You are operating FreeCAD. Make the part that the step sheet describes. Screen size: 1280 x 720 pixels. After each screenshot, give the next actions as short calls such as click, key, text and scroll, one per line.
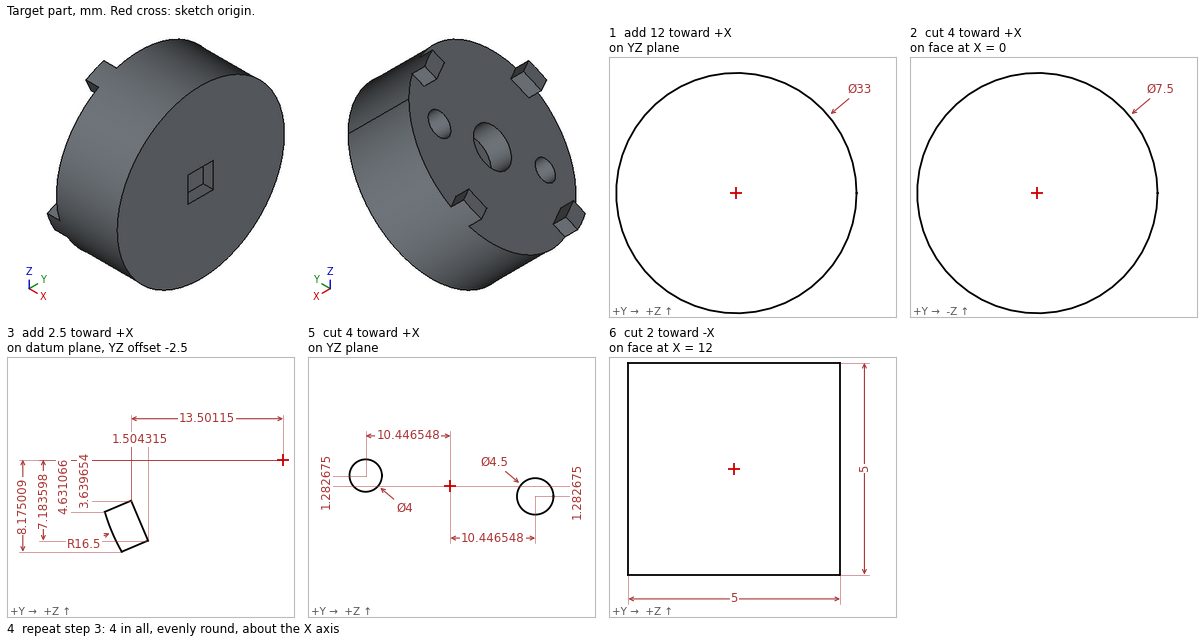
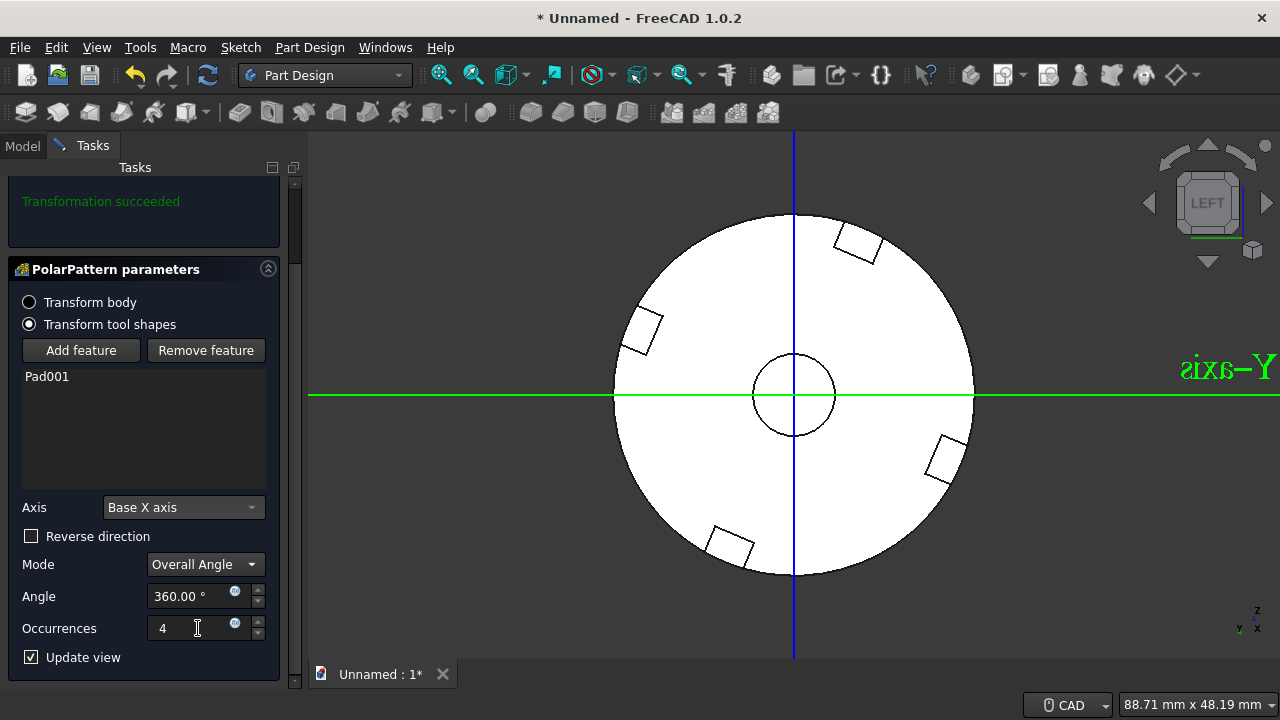
scroll(295, 432, up, 3)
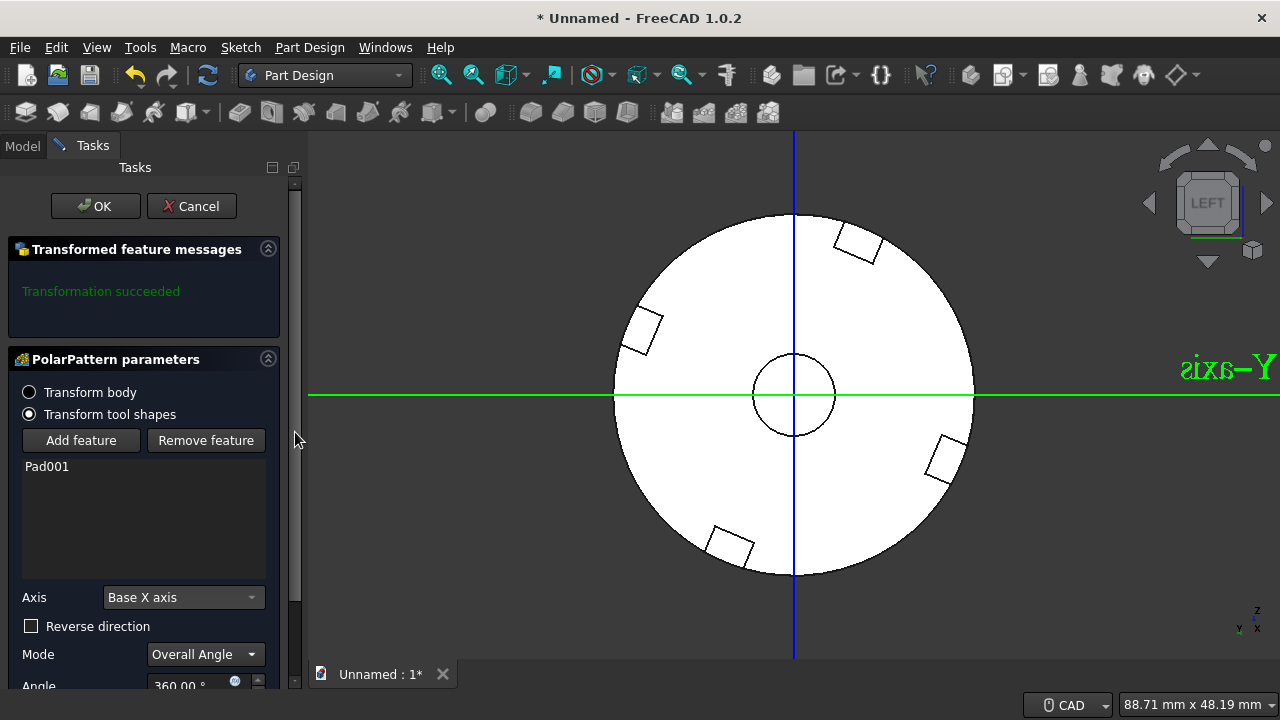
click(96, 206)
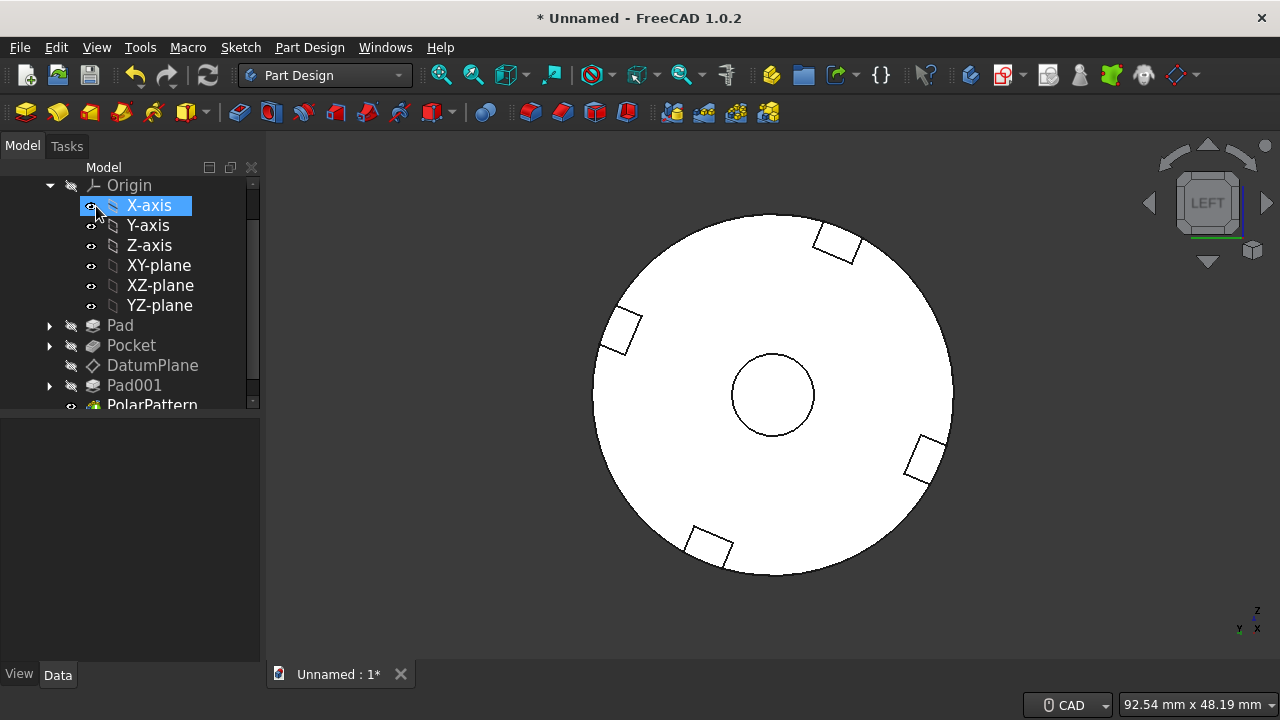
click(1004, 76)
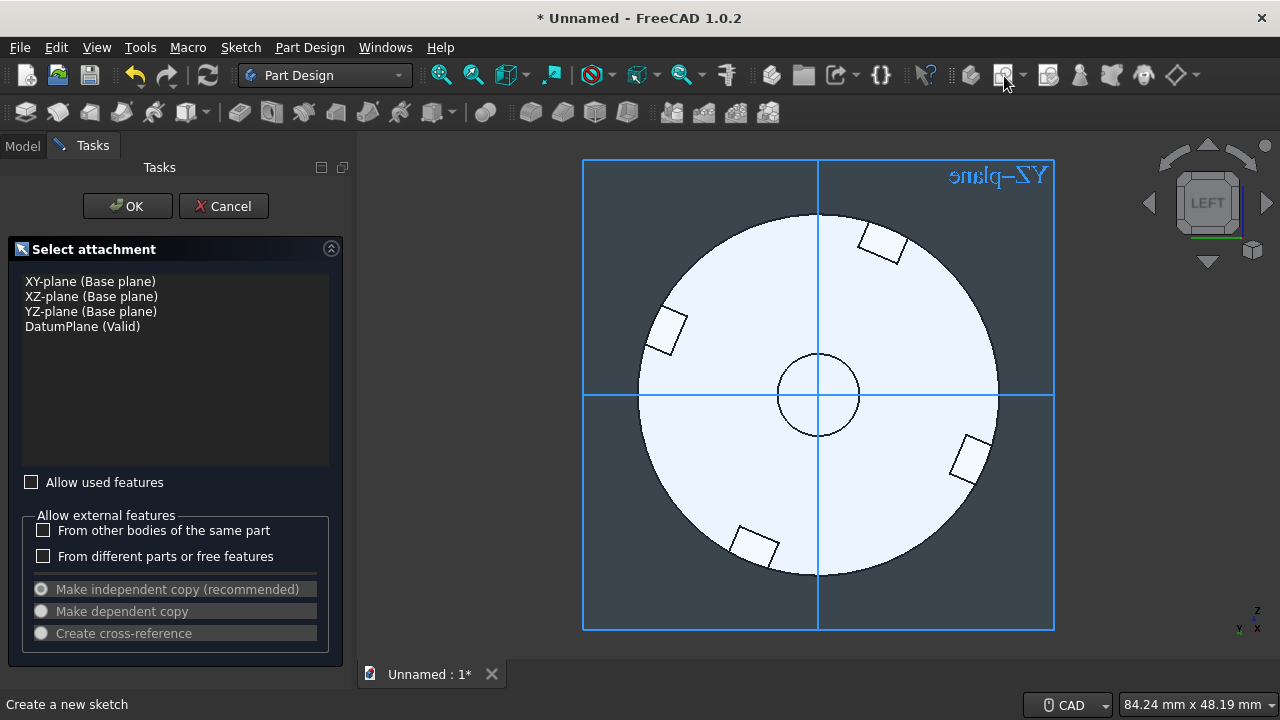
click(82, 312)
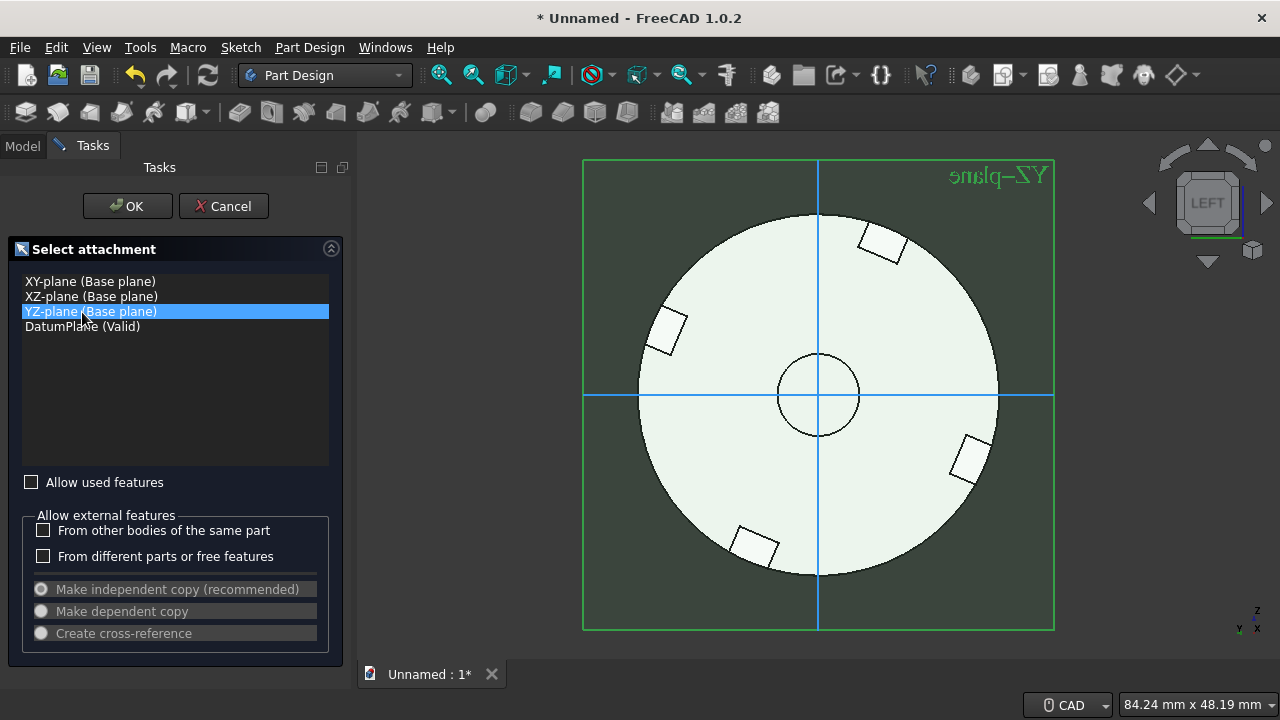
click(128, 206)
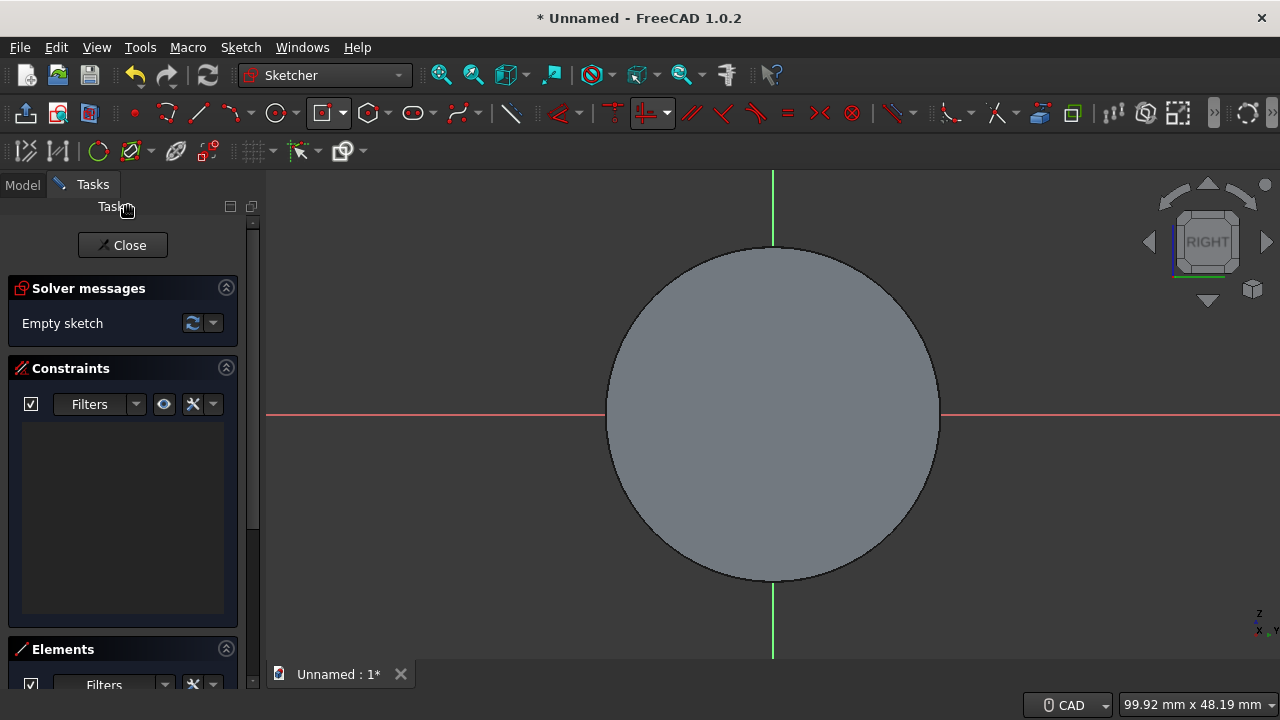
key(q)
key(s)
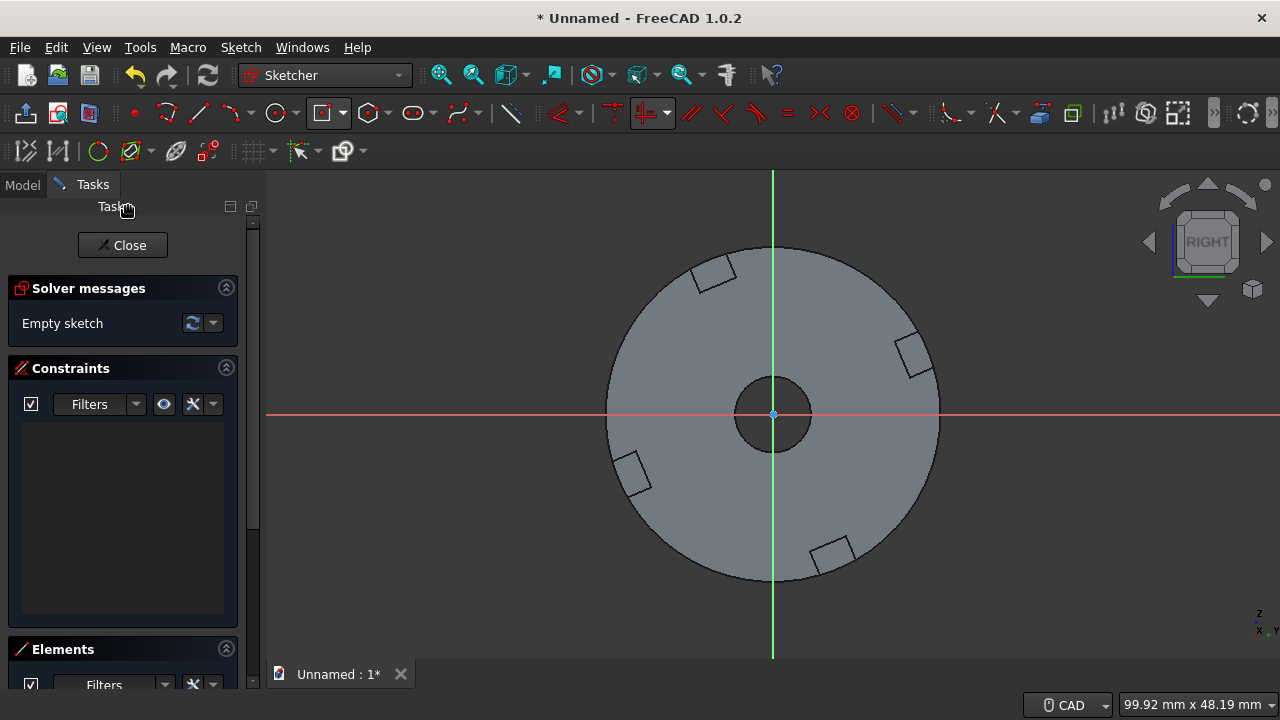
scroll(831, 417, up, 4)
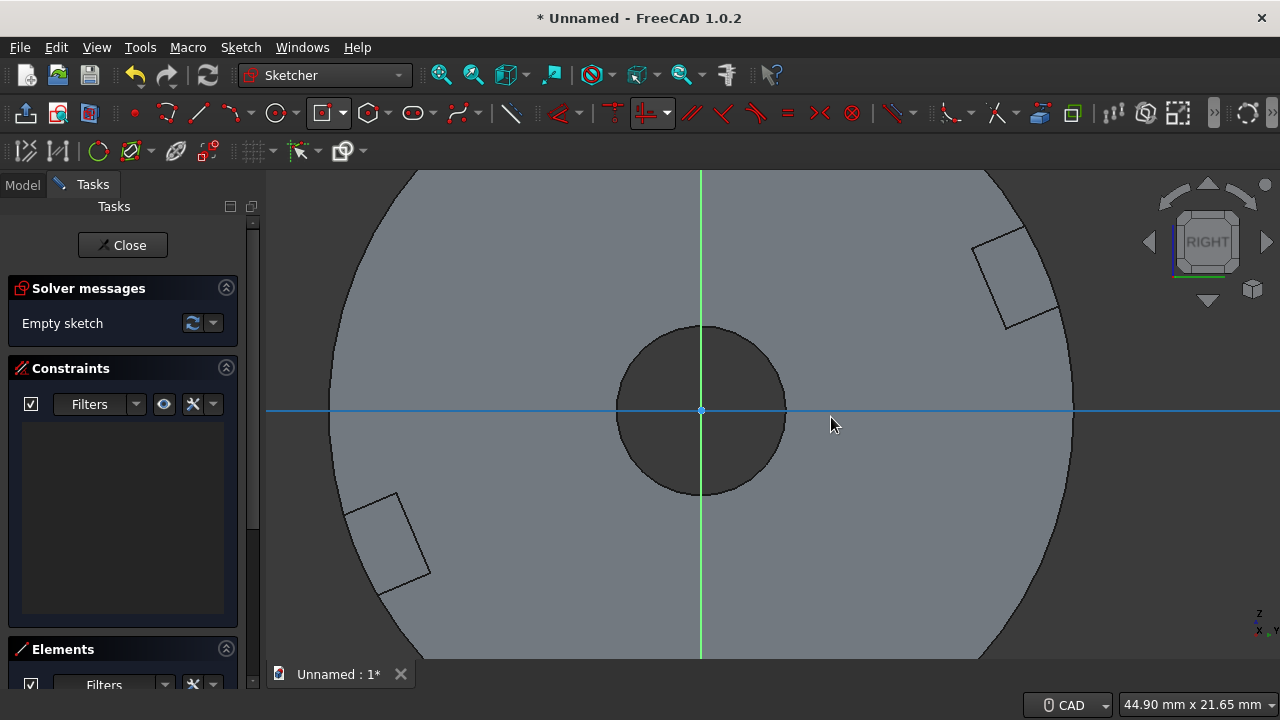
key(g)
key(c)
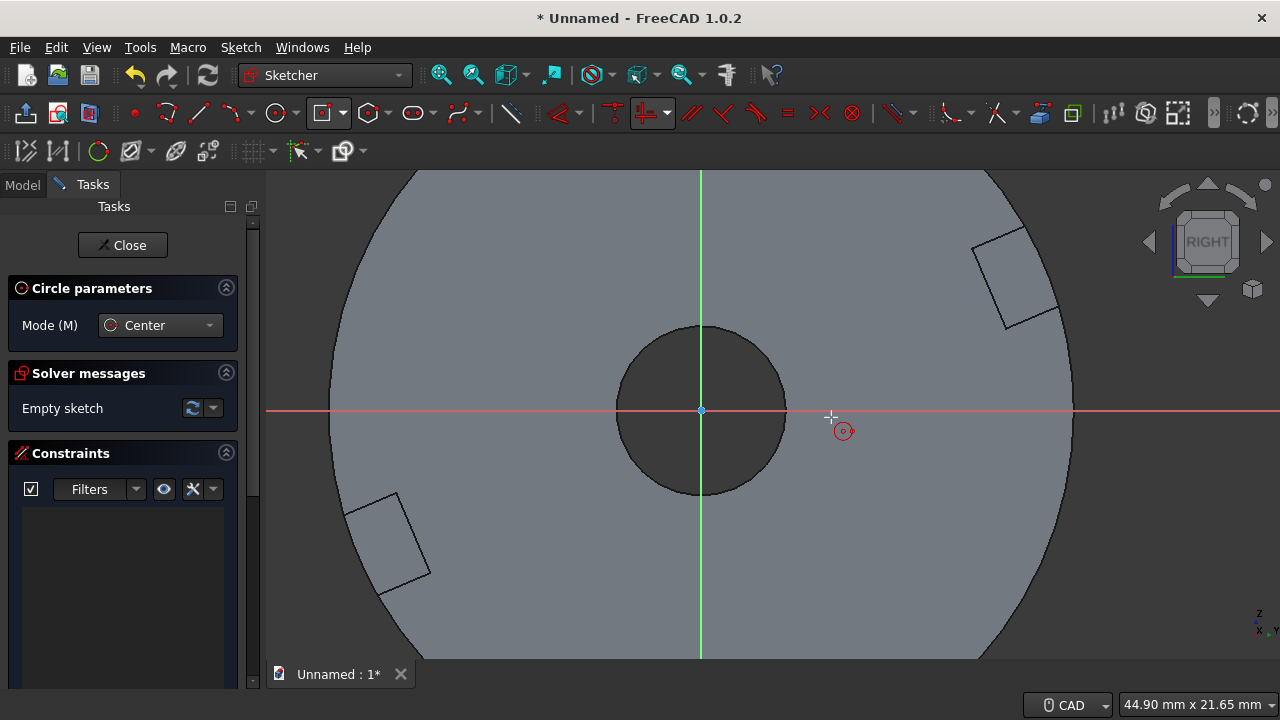
click(937, 440)
click(973, 476)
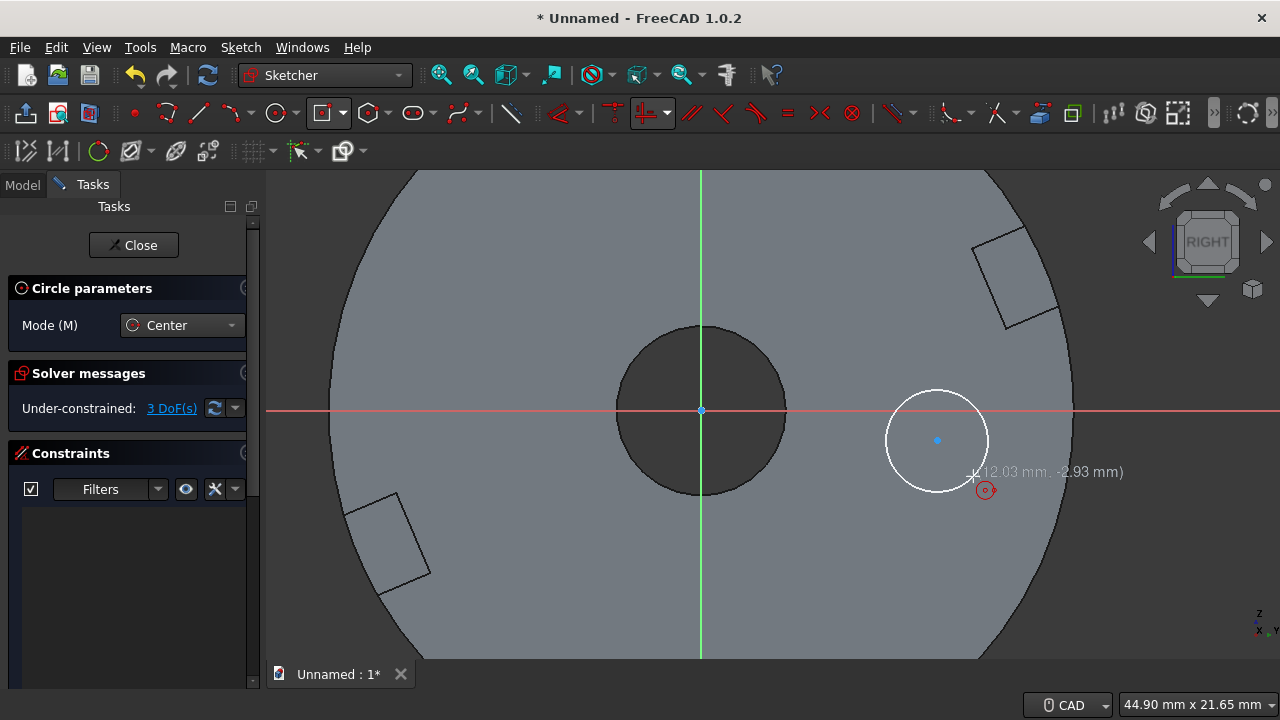
click(465, 382)
click(497, 350)
key(Escape)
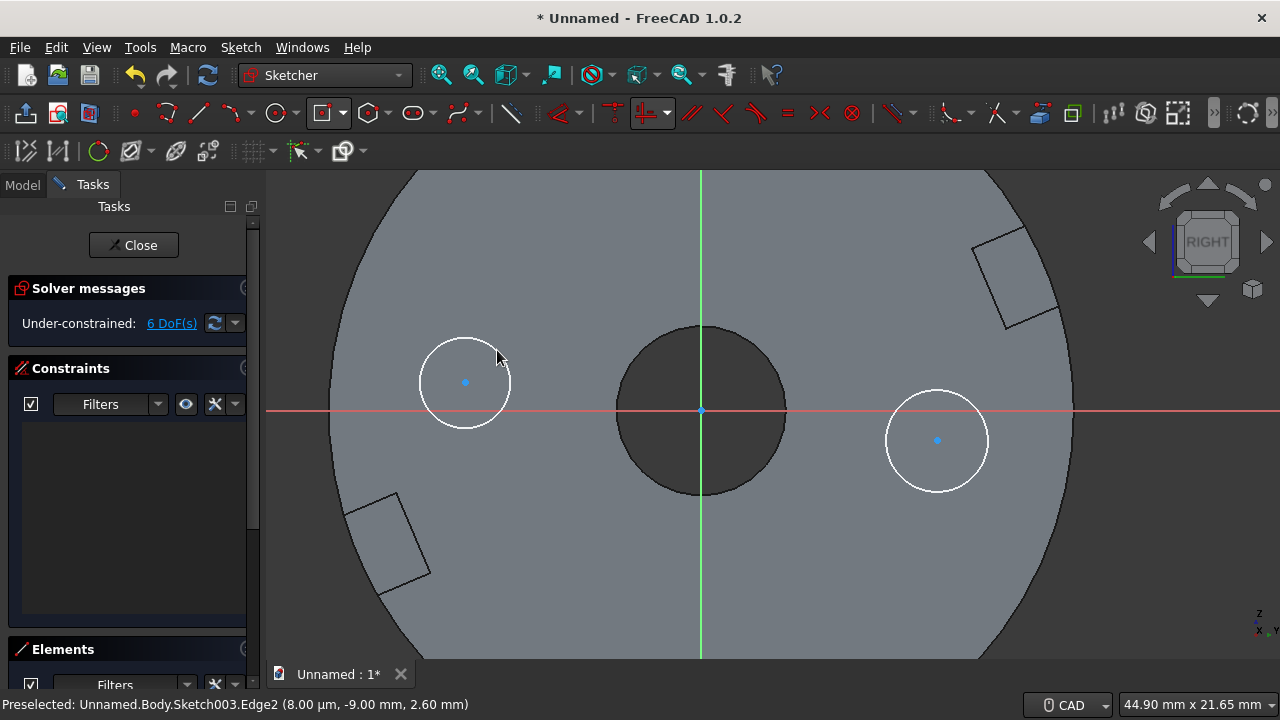
key(d)